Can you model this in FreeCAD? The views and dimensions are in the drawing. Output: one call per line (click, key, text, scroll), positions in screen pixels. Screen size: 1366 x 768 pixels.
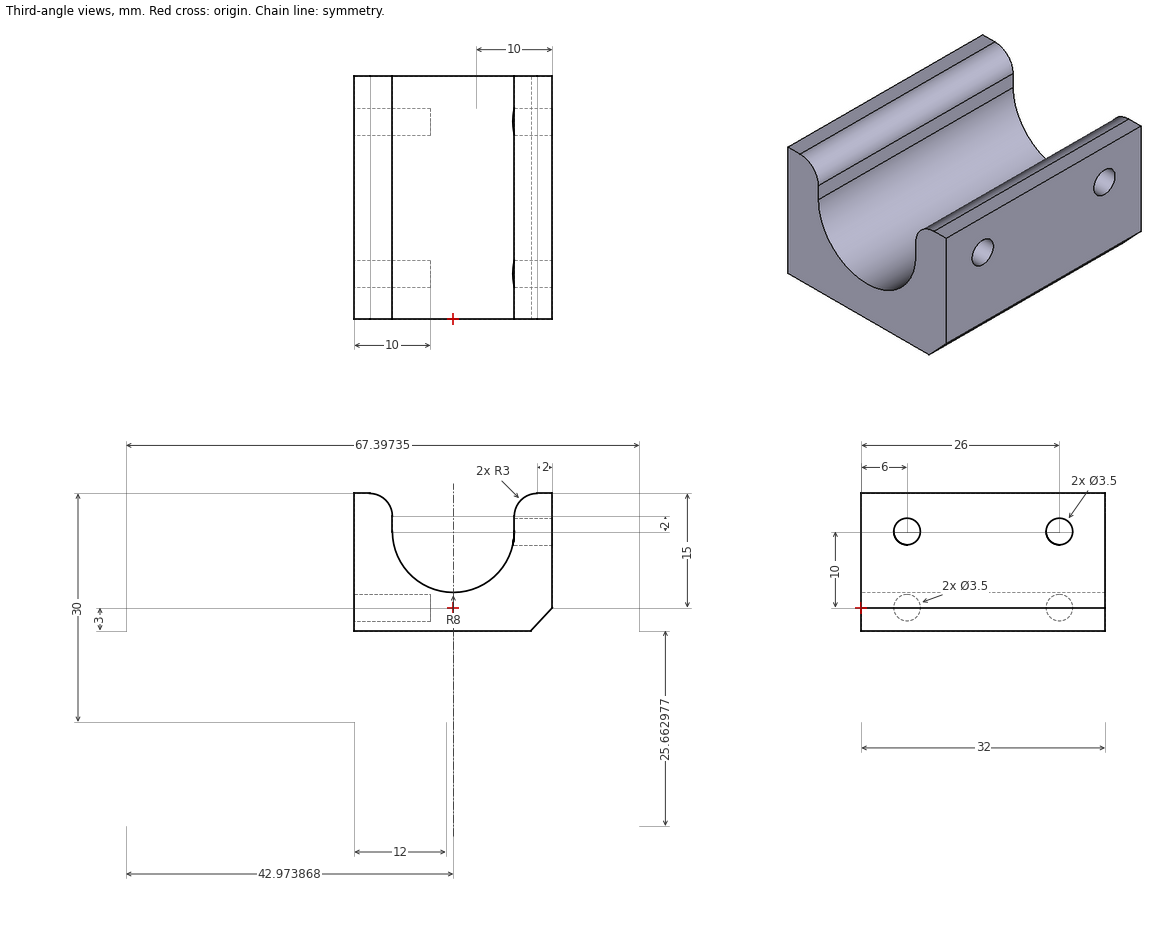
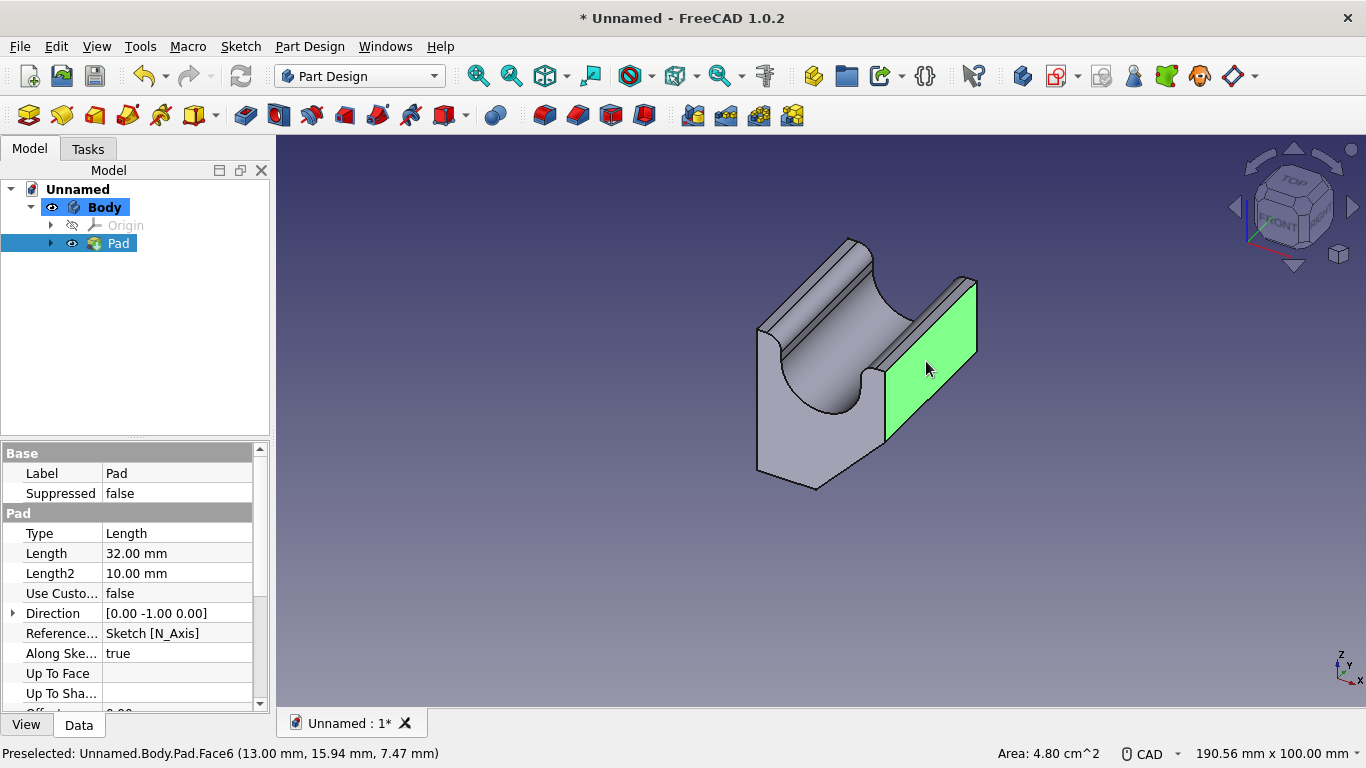
click(1056, 76)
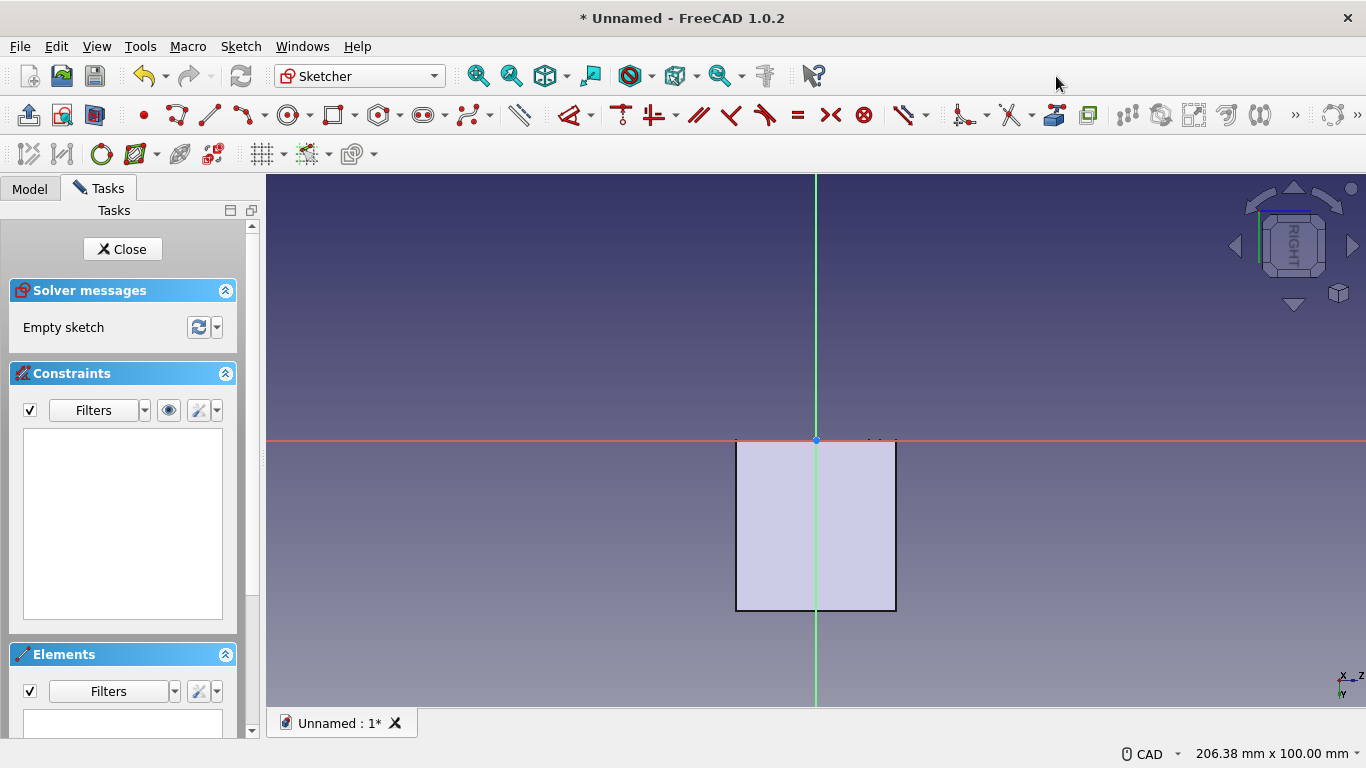
scroll(929, 575, up, 4)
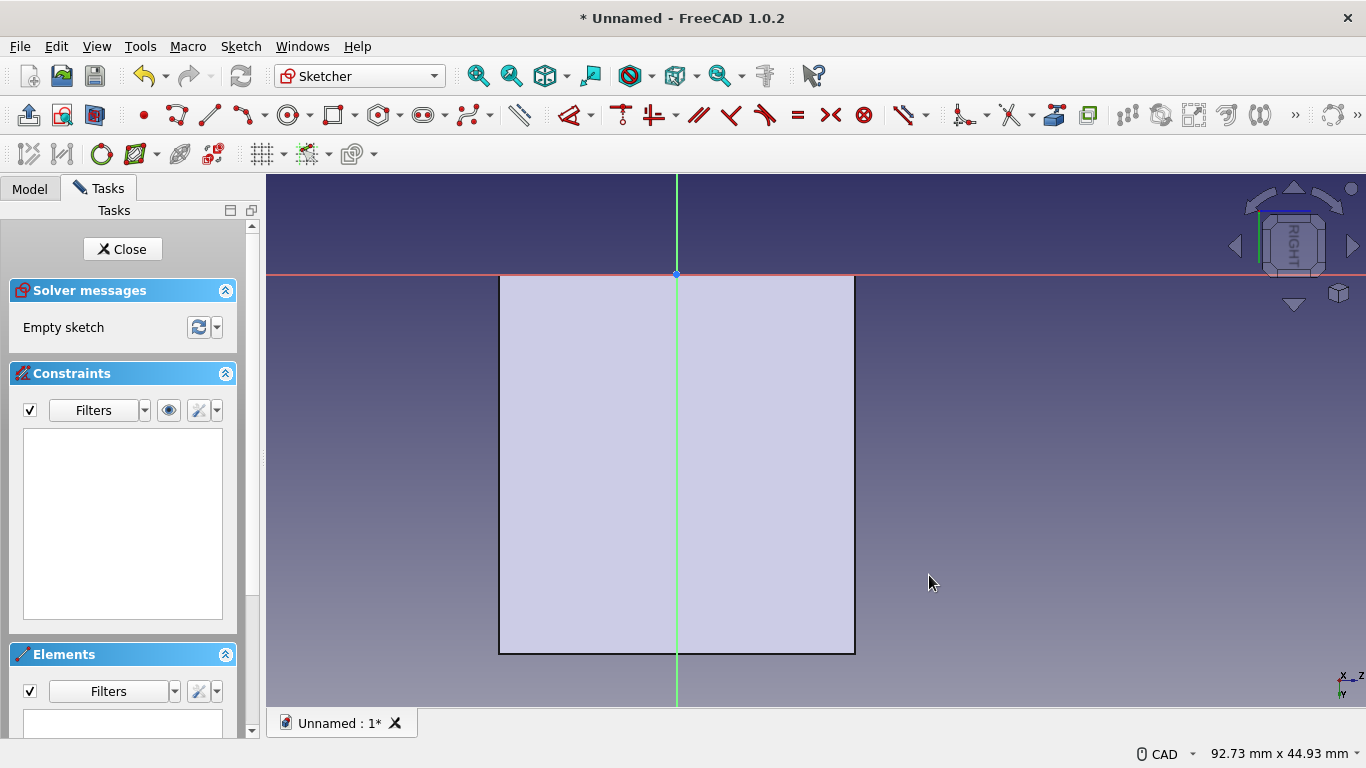
click(288, 116)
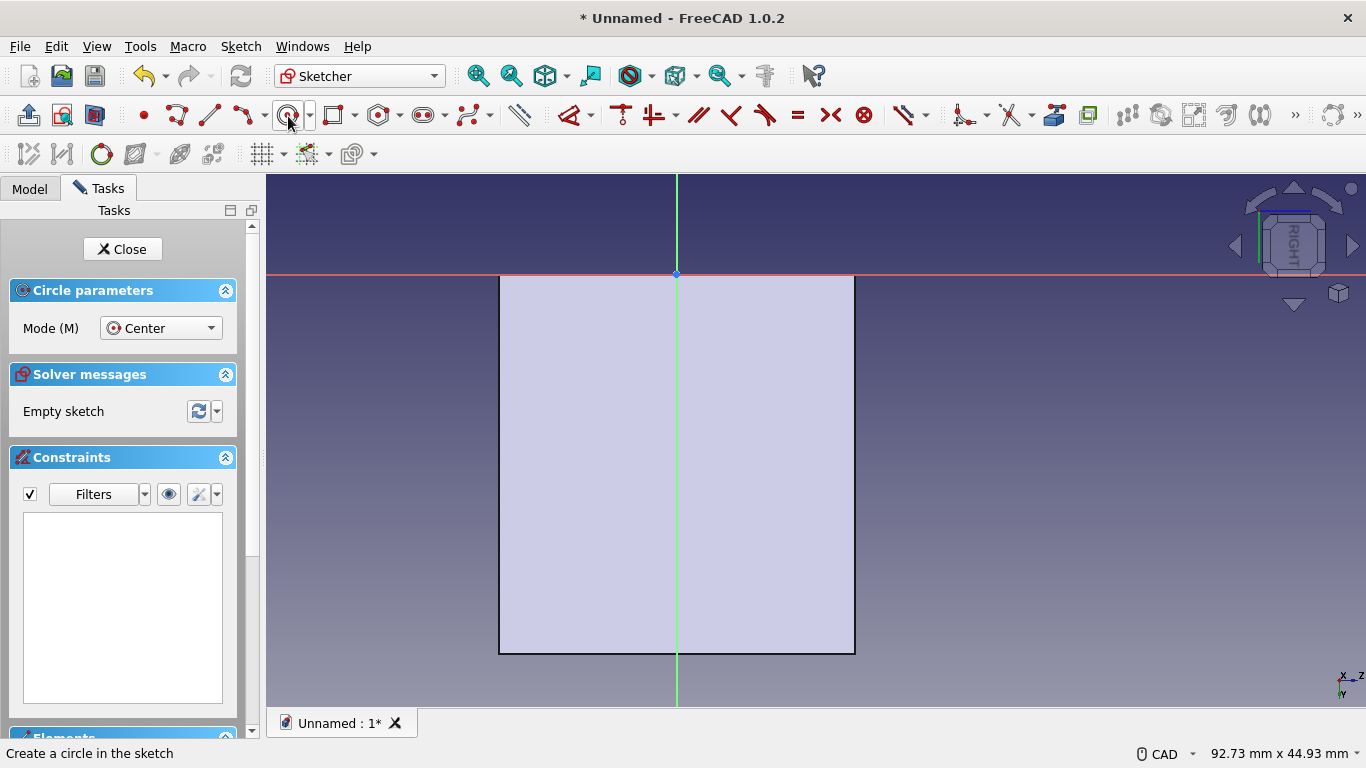
click(795, 583)
move(810, 568)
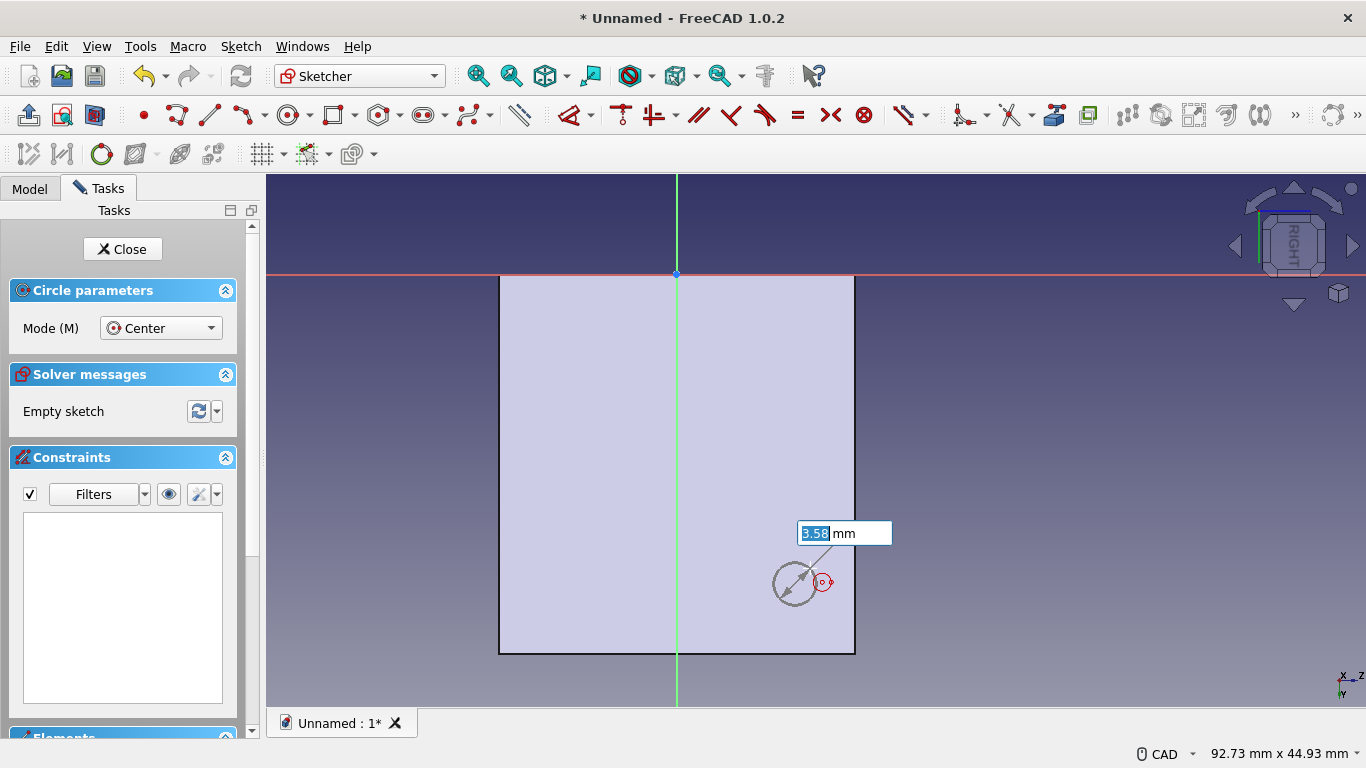
text(3.5)
key(Return)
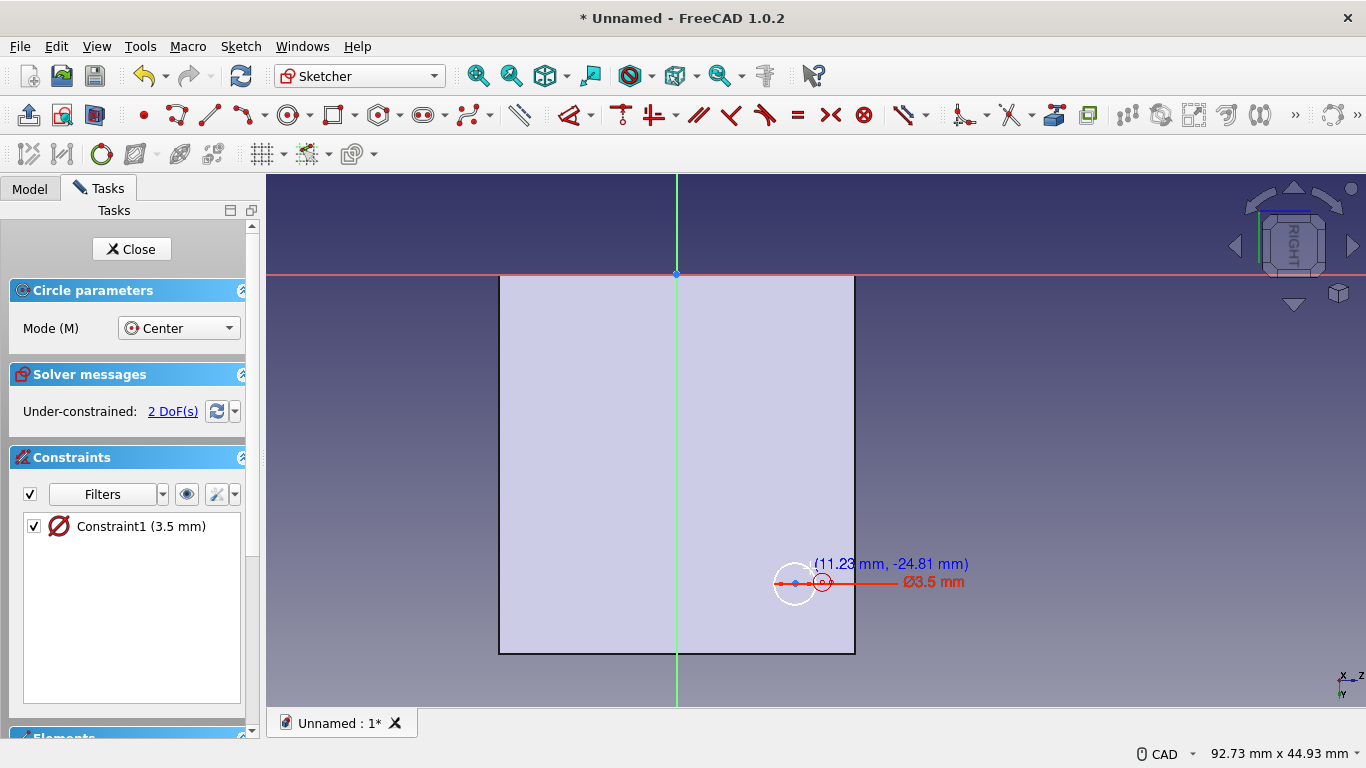
click(795, 346)
move(810, 331)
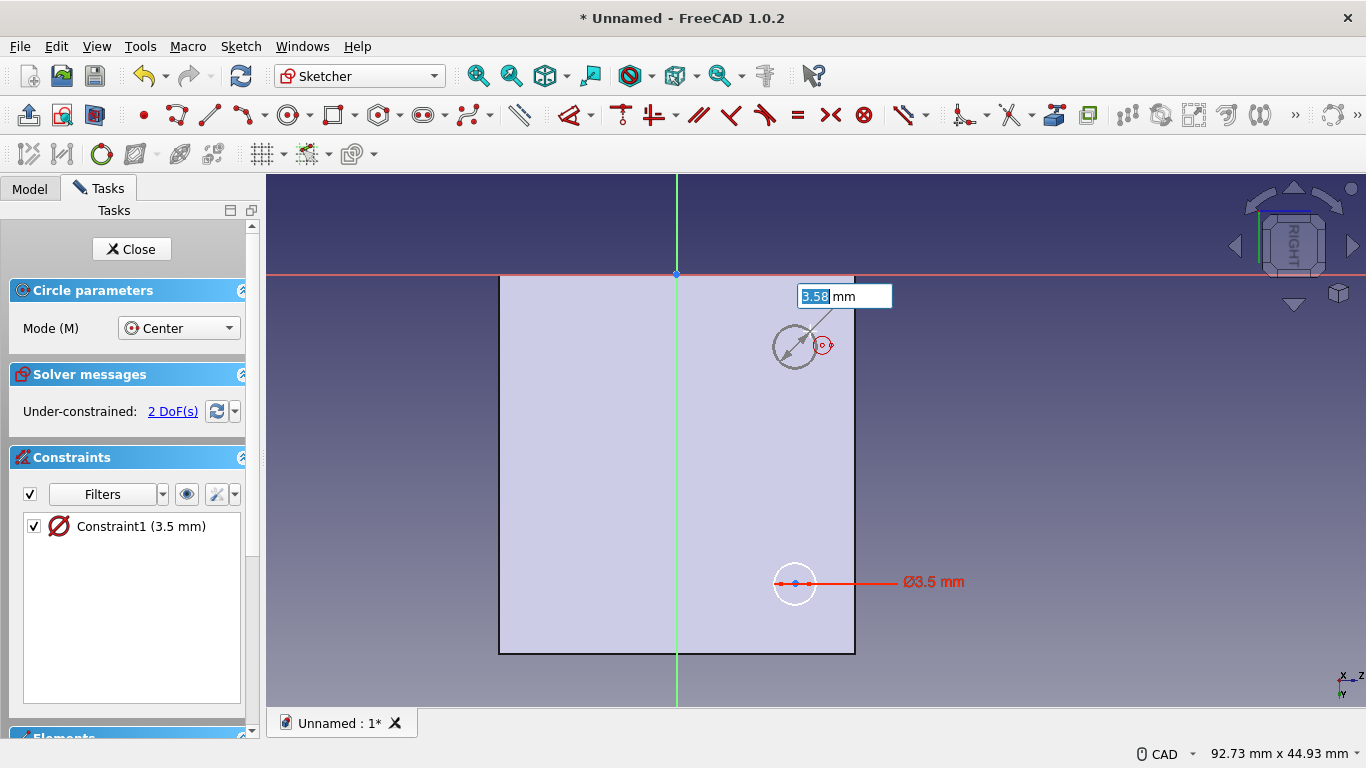
text(3.5)
key(Return)
key(Escape)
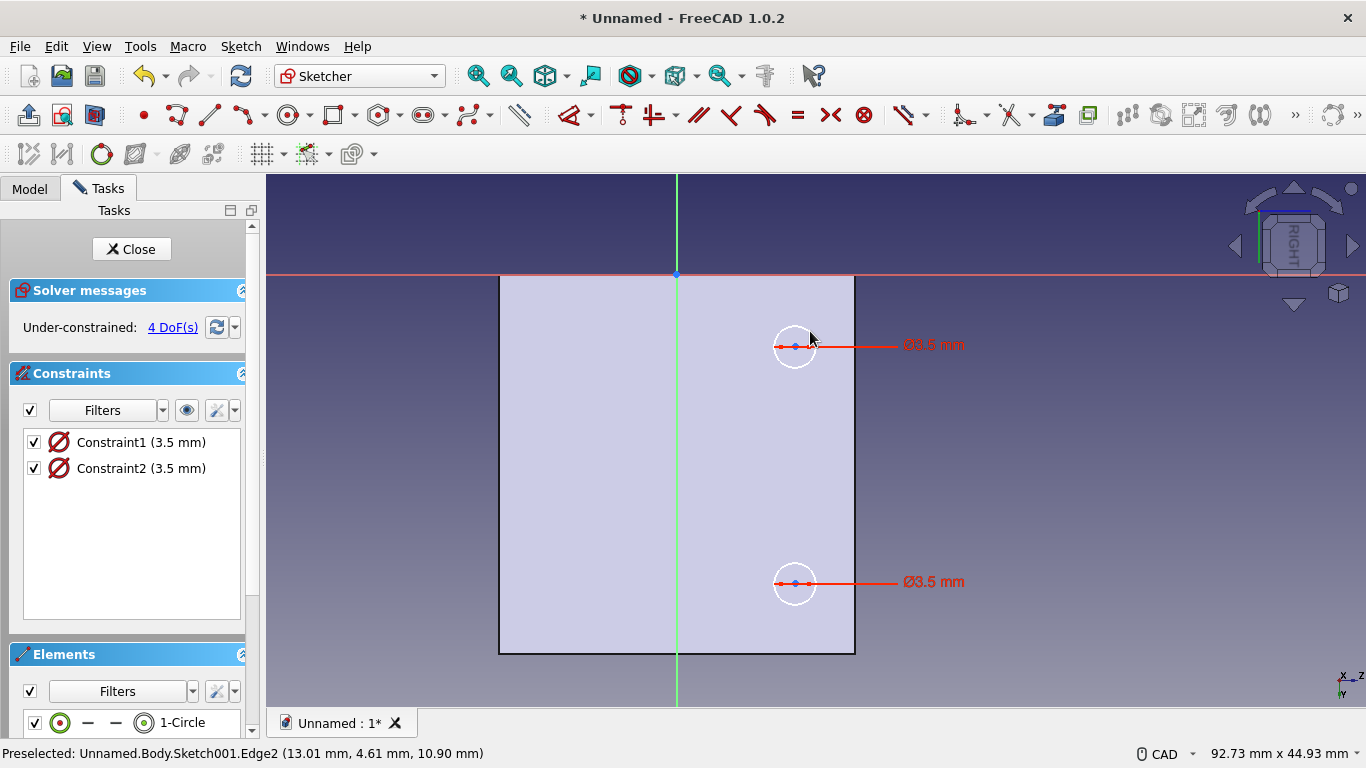
click(568, 116)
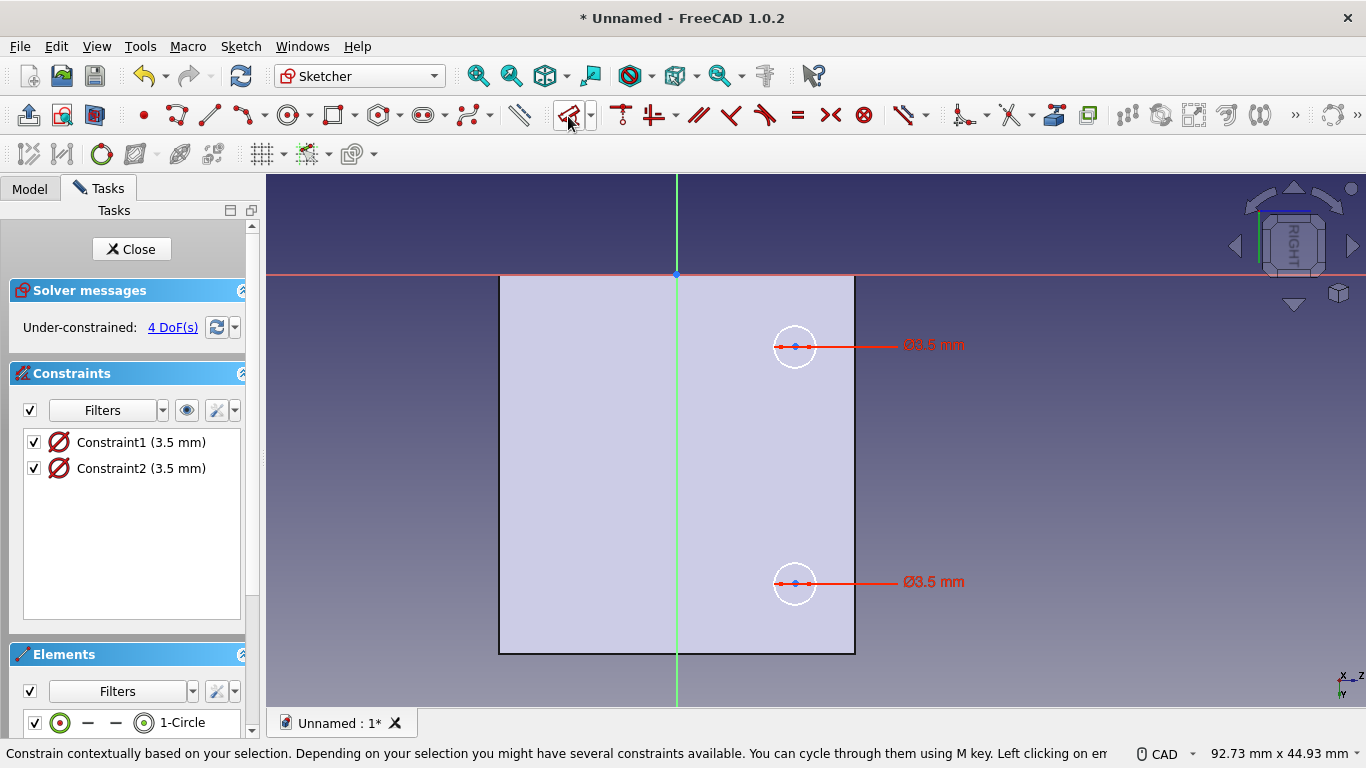
click(795, 347)
click(643, 311)